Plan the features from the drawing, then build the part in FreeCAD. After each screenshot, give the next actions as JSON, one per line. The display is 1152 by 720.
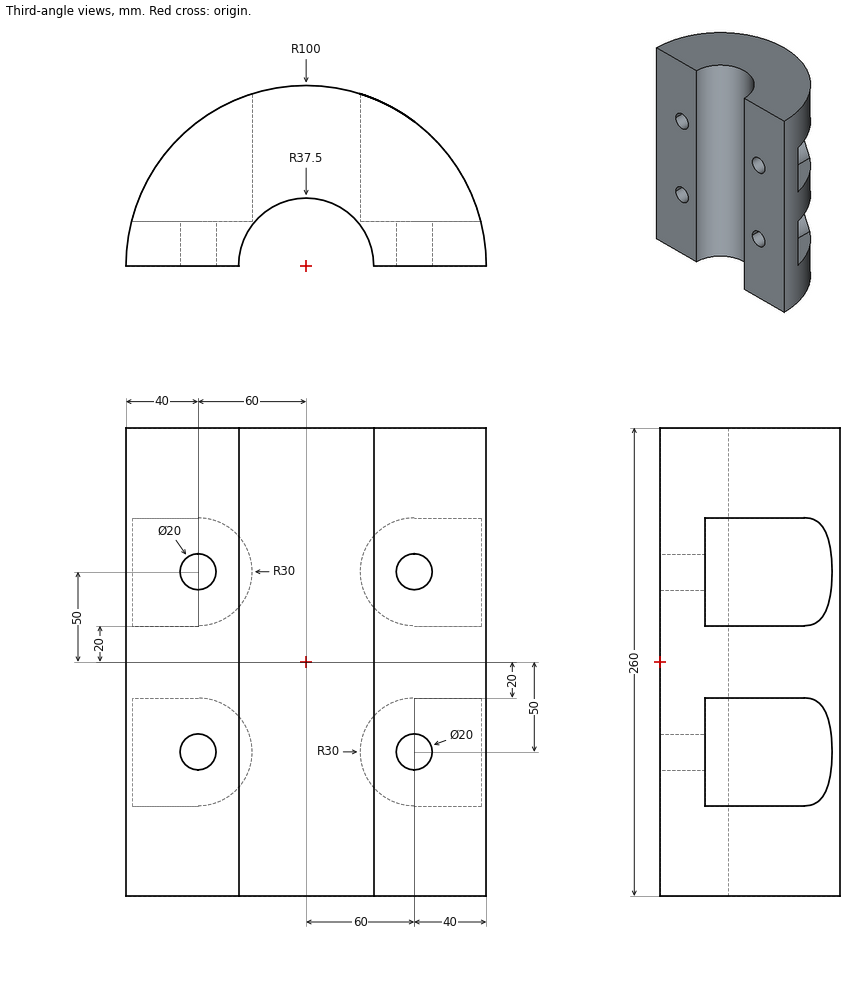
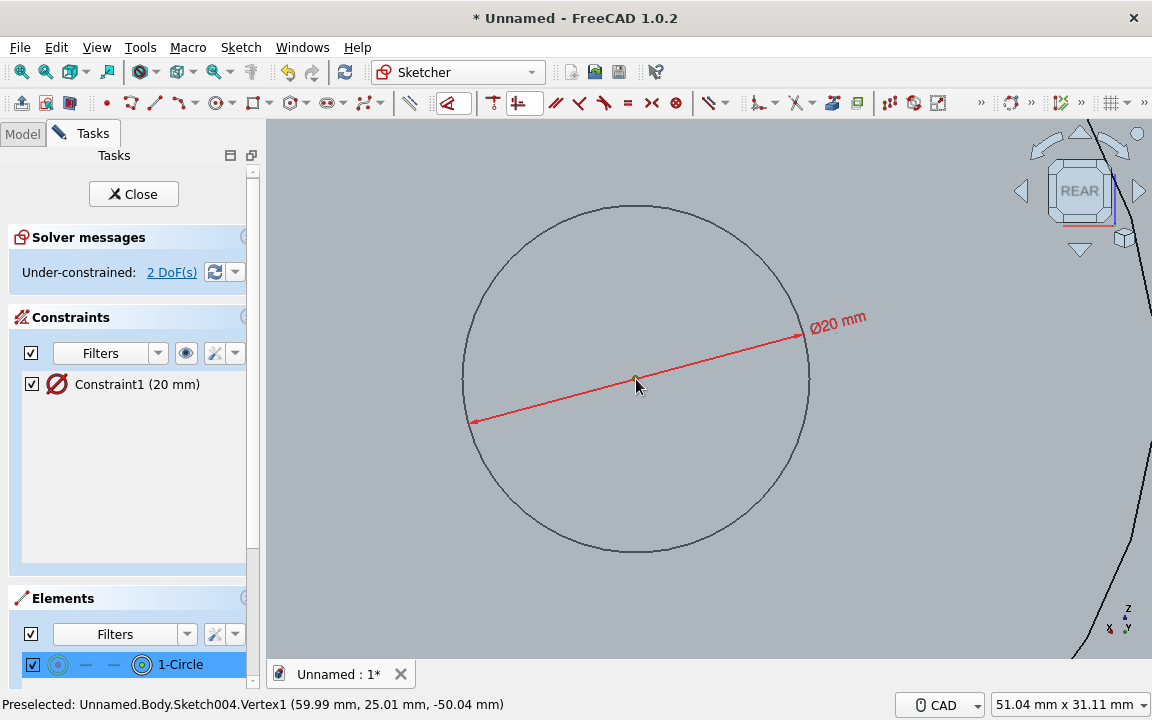
{"action": "left_click", "coordinate": [466, 104]}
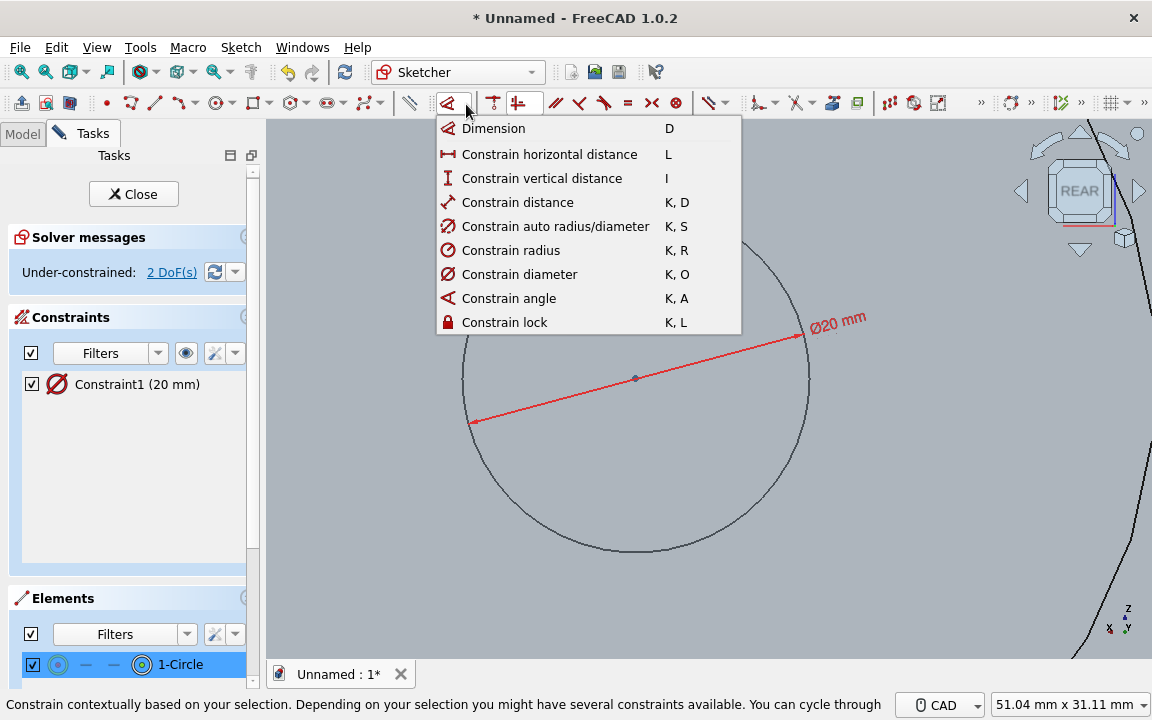
{"action": "left_click", "coordinate": [589, 154]}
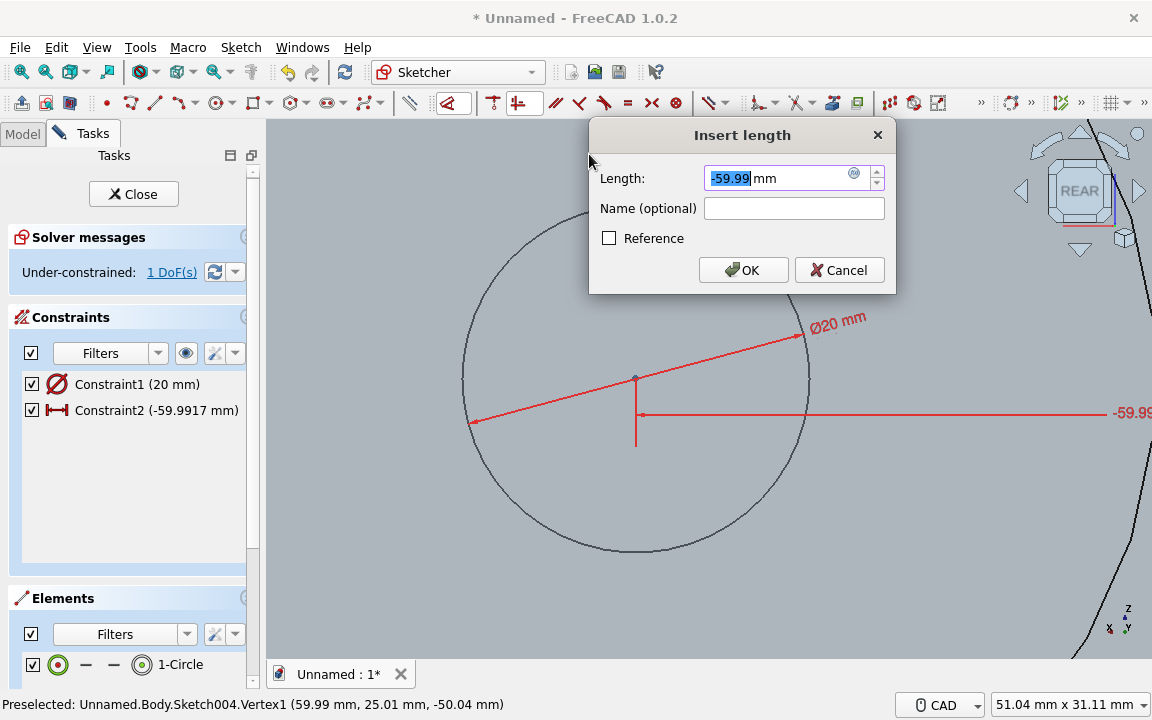
{"action": "type", "text": "-60"}
{"action": "key", "text": "Return"}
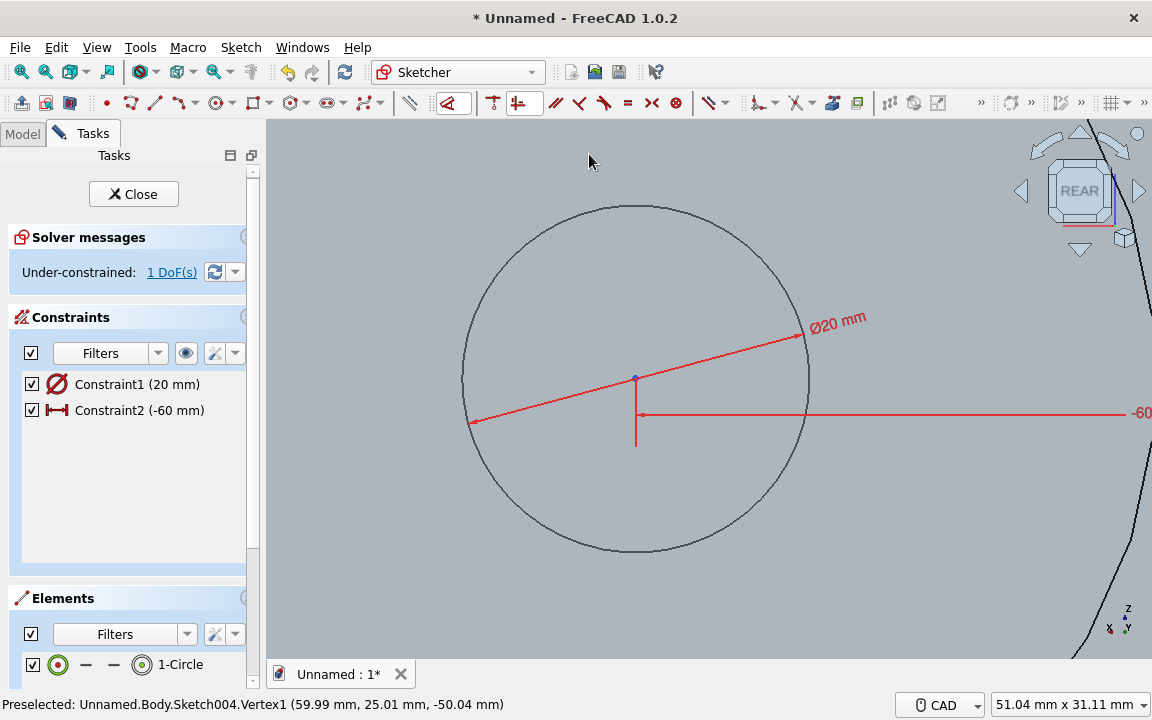
{"action": "left_click", "coordinate": [636, 379]}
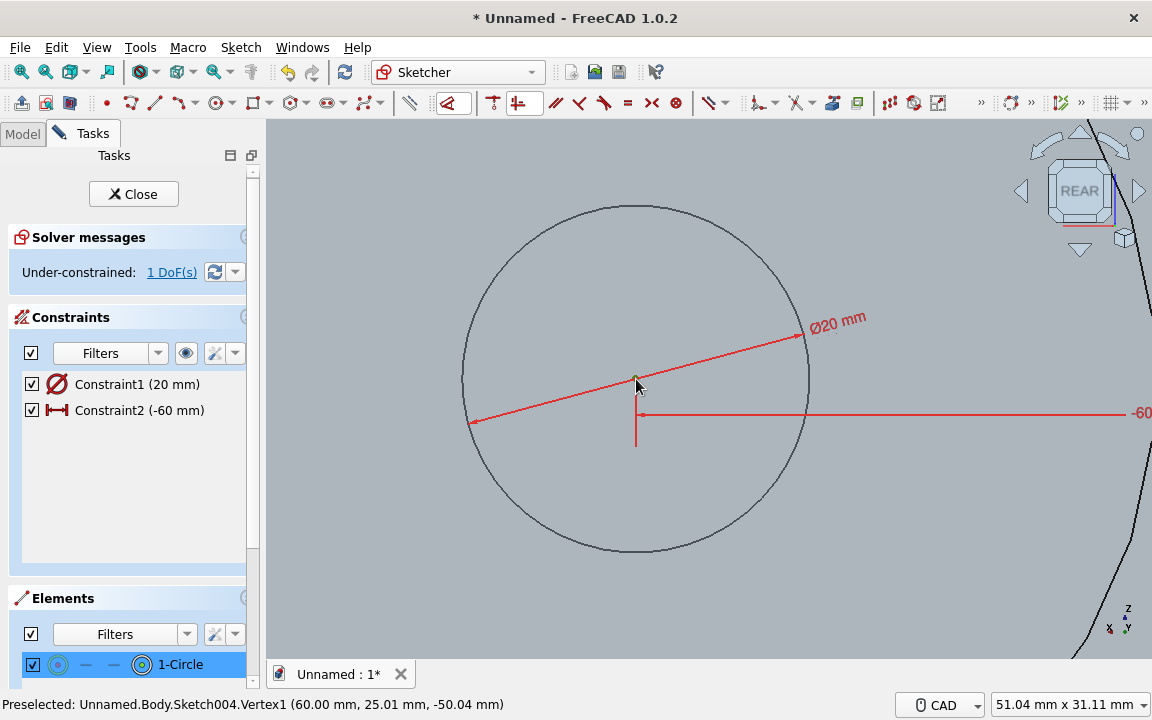
{"action": "left_click", "coordinate": [466, 104]}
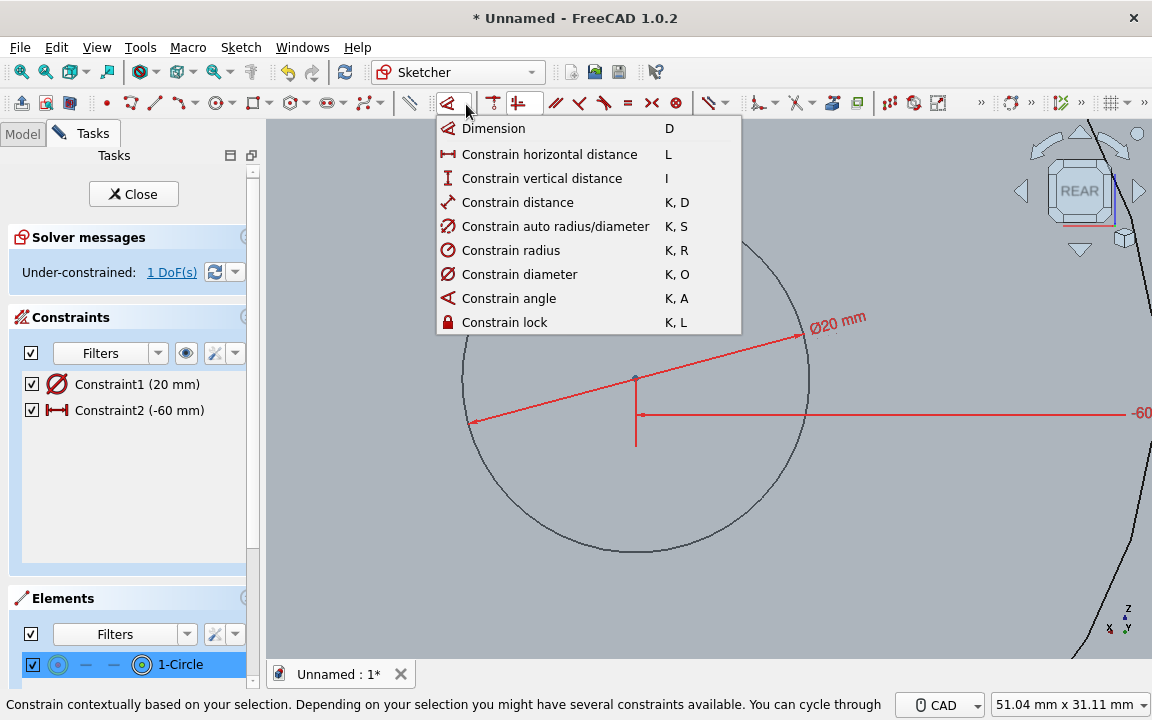
{"action": "left_click", "coordinate": [589, 178]}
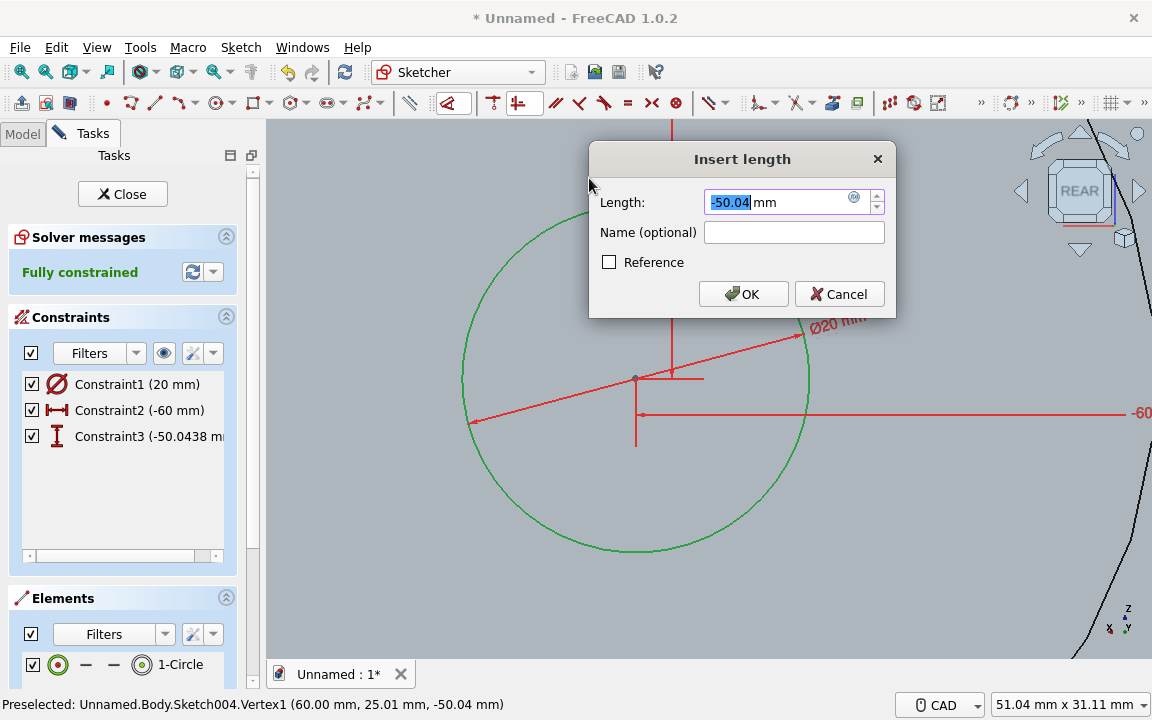
{"action": "type", "text": "-50"}
{"action": "key", "text": "Return"}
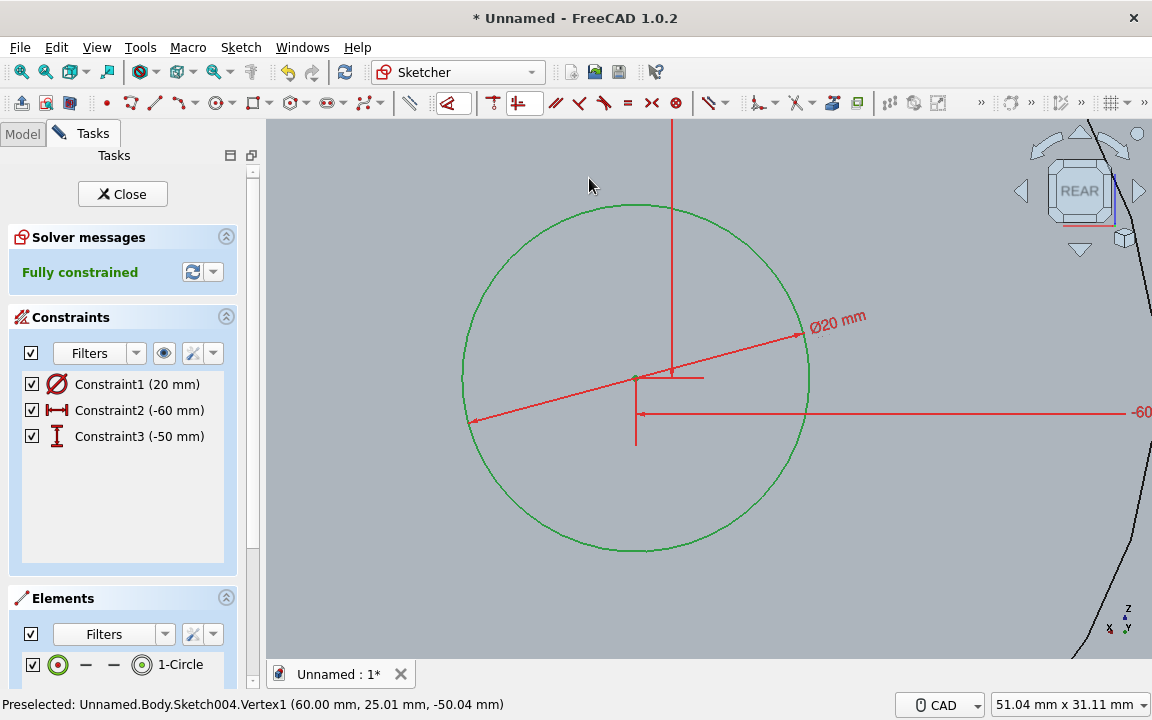
{"action": "left_click", "coordinate": [123, 194]}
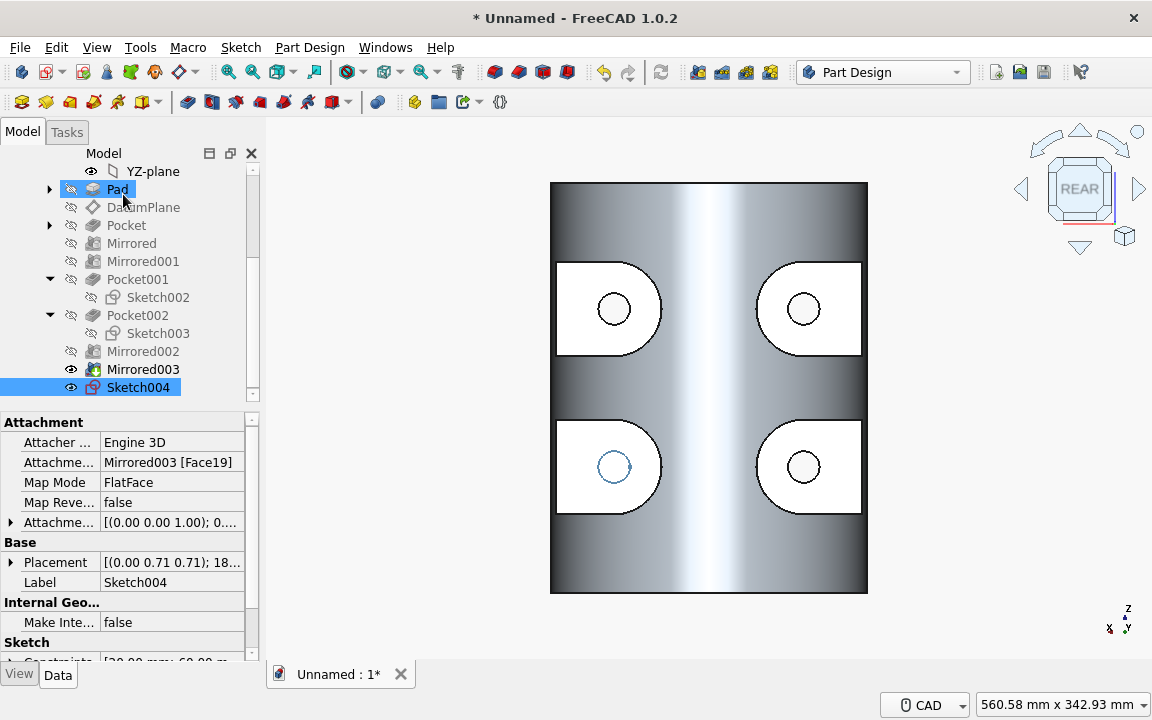
{"action": "left_click", "coordinate": [188, 102]}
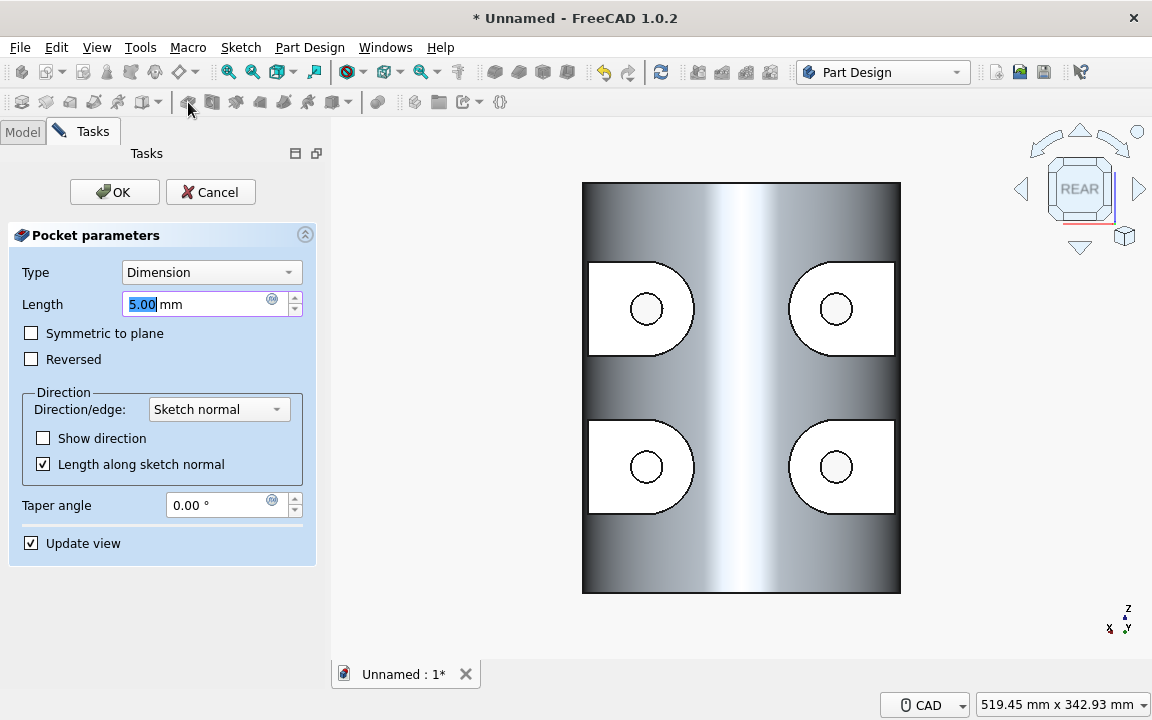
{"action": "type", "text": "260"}
{"action": "key", "text": "Tab"}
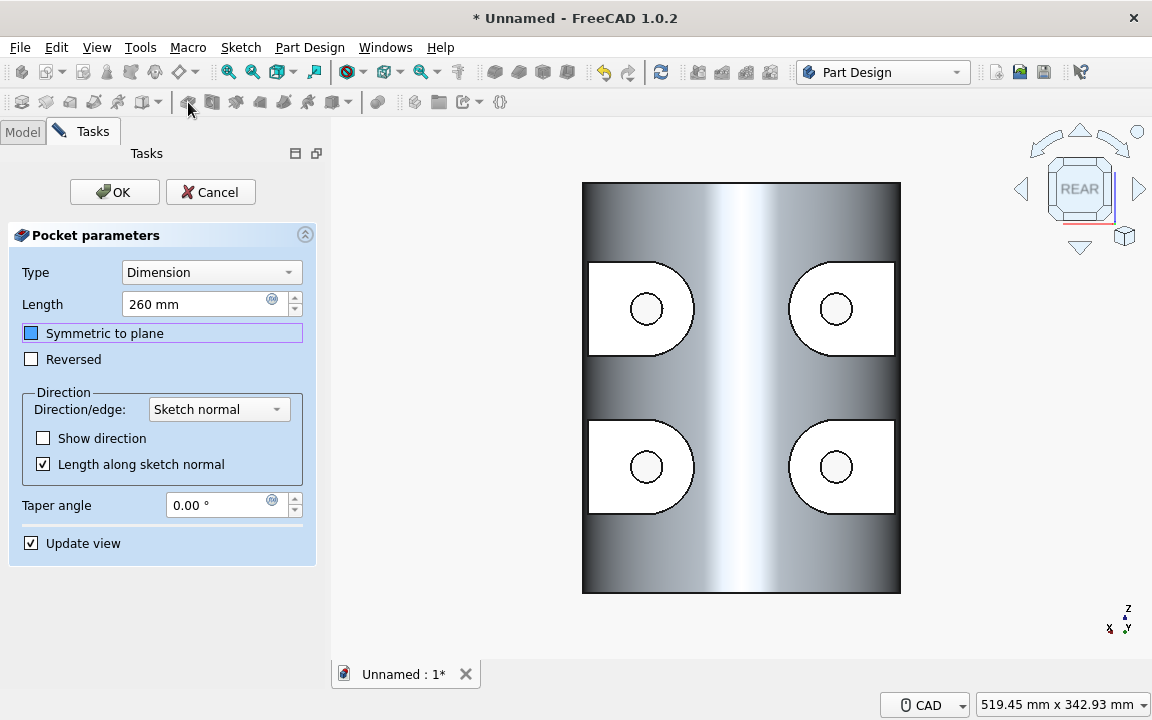
{"action": "left_click", "coordinate": [115, 192]}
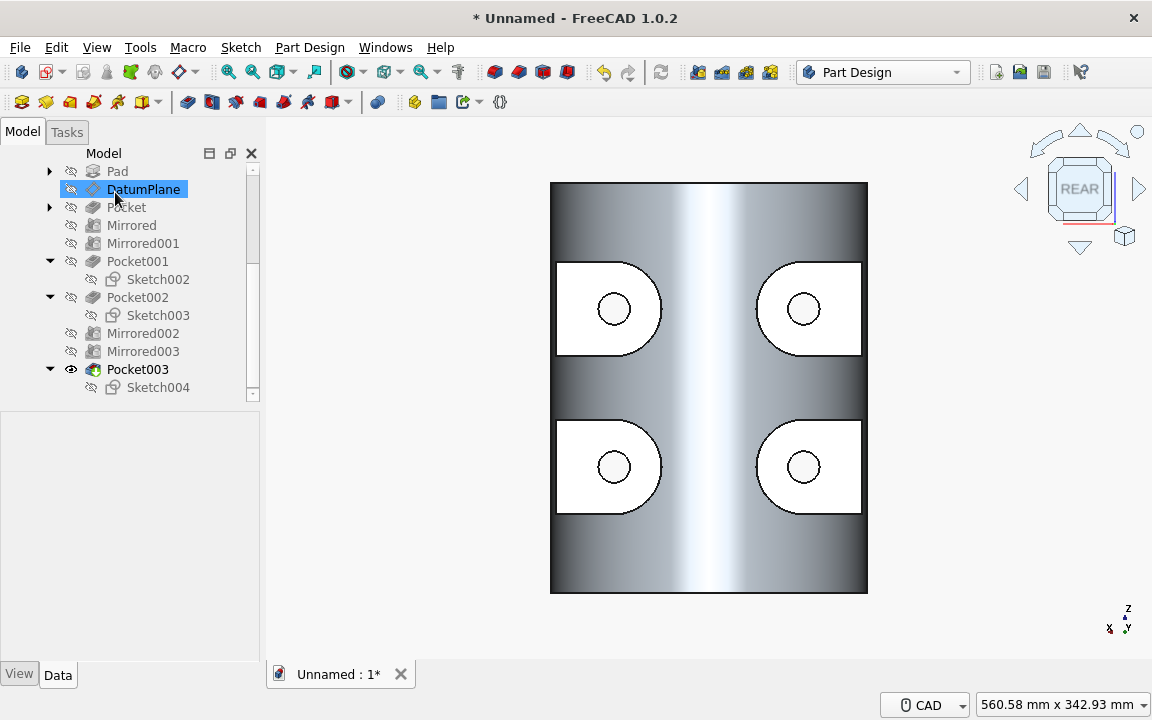
{"action": "key", "text": "0"}